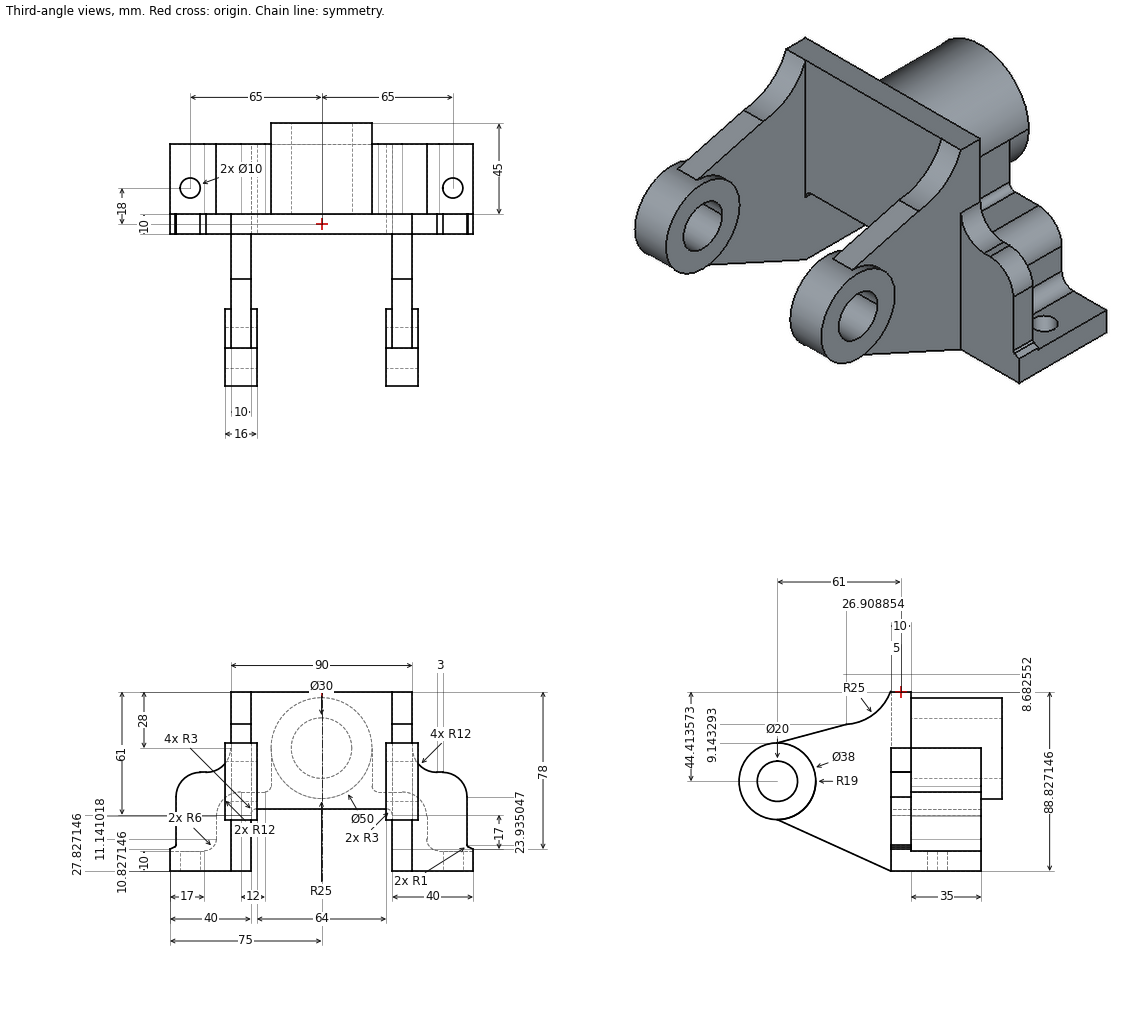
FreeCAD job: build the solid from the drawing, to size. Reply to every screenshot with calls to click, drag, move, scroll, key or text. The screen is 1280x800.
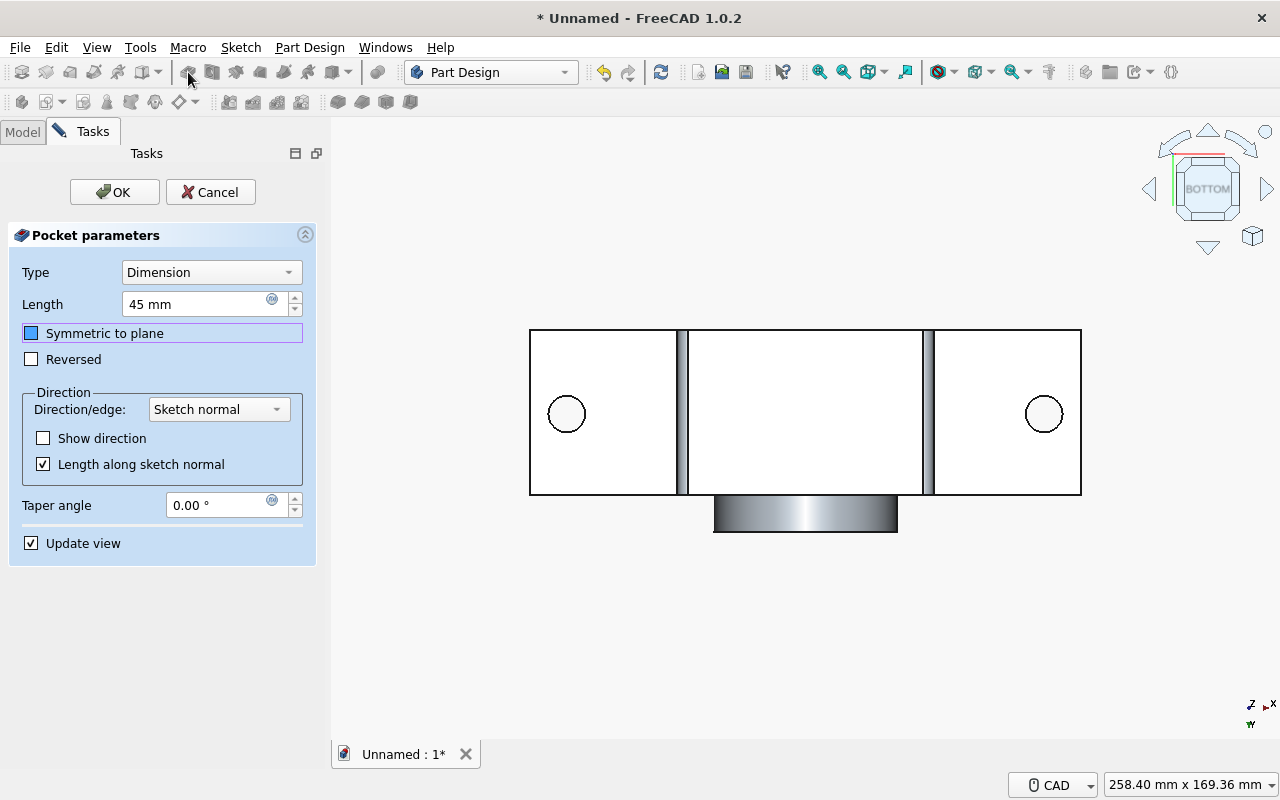
click(30, 333)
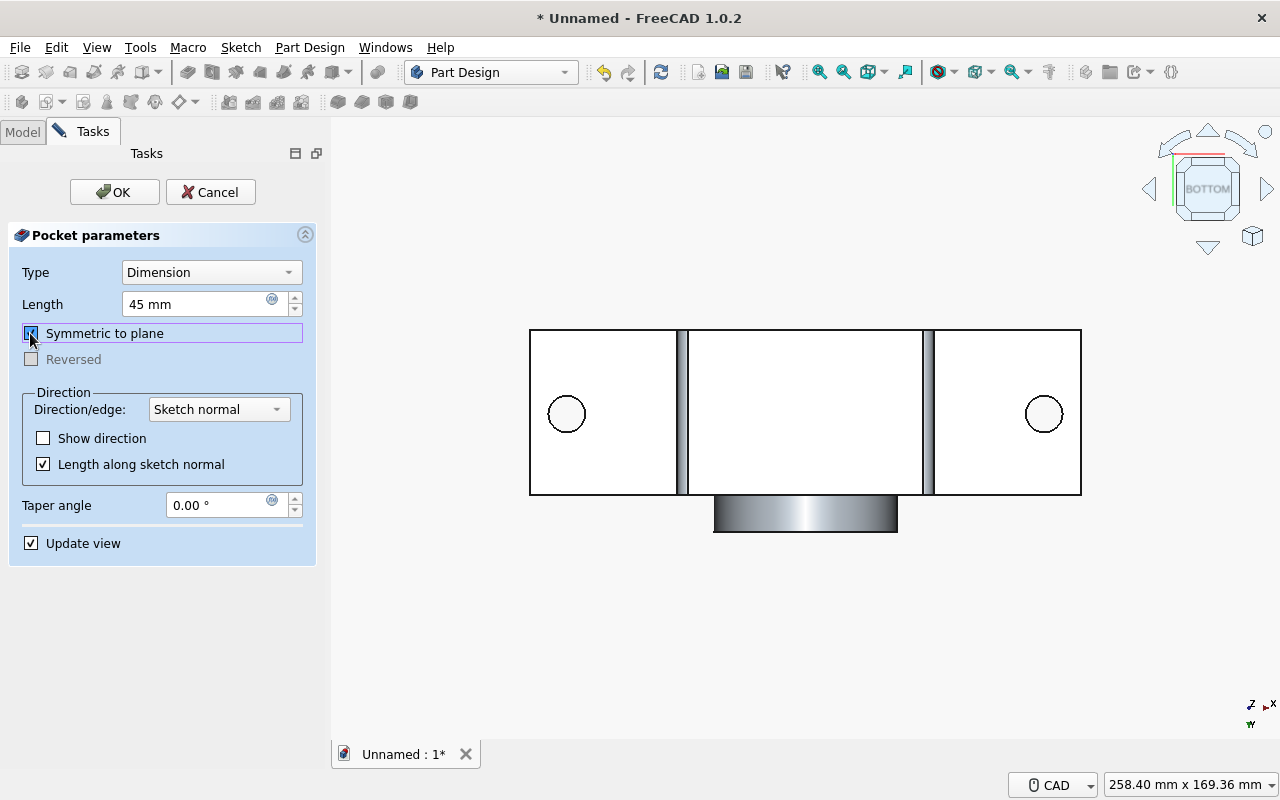
click(115, 192)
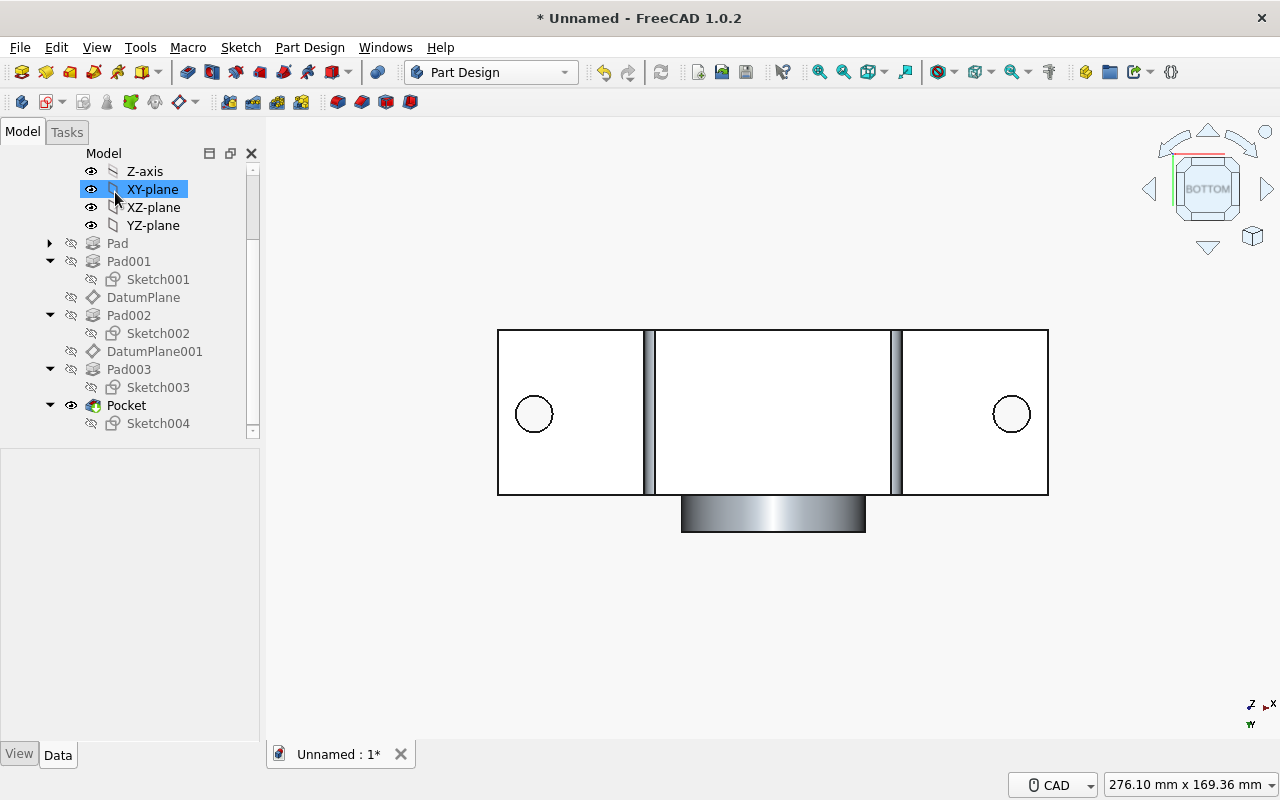
key(6)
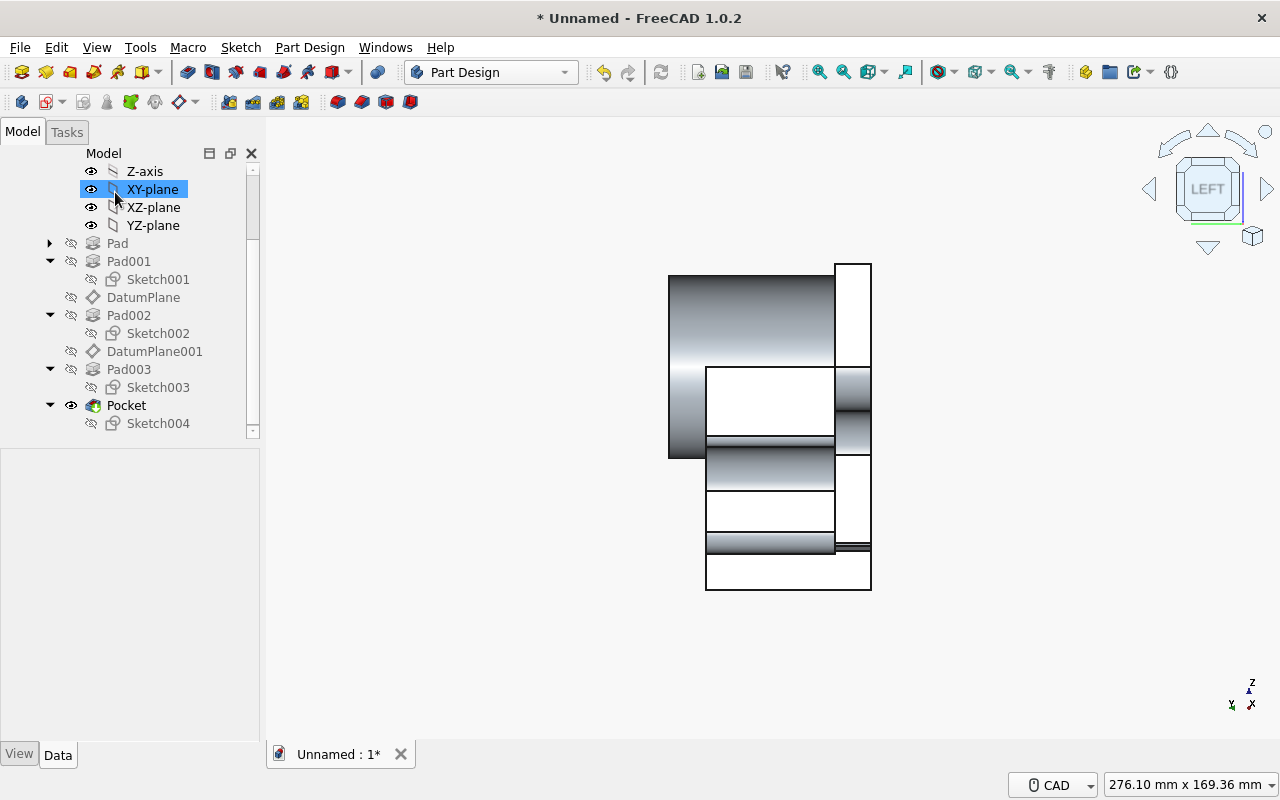
click(853, 285)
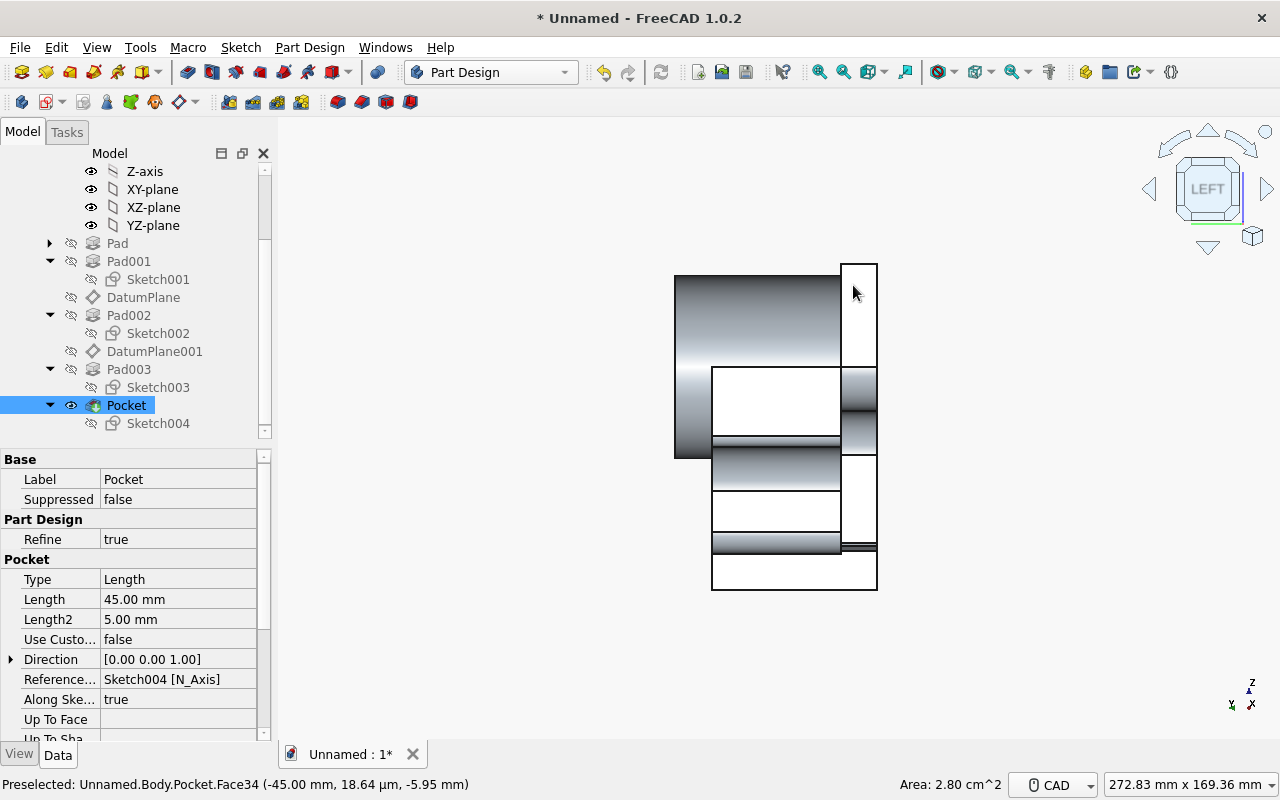
click(46, 102)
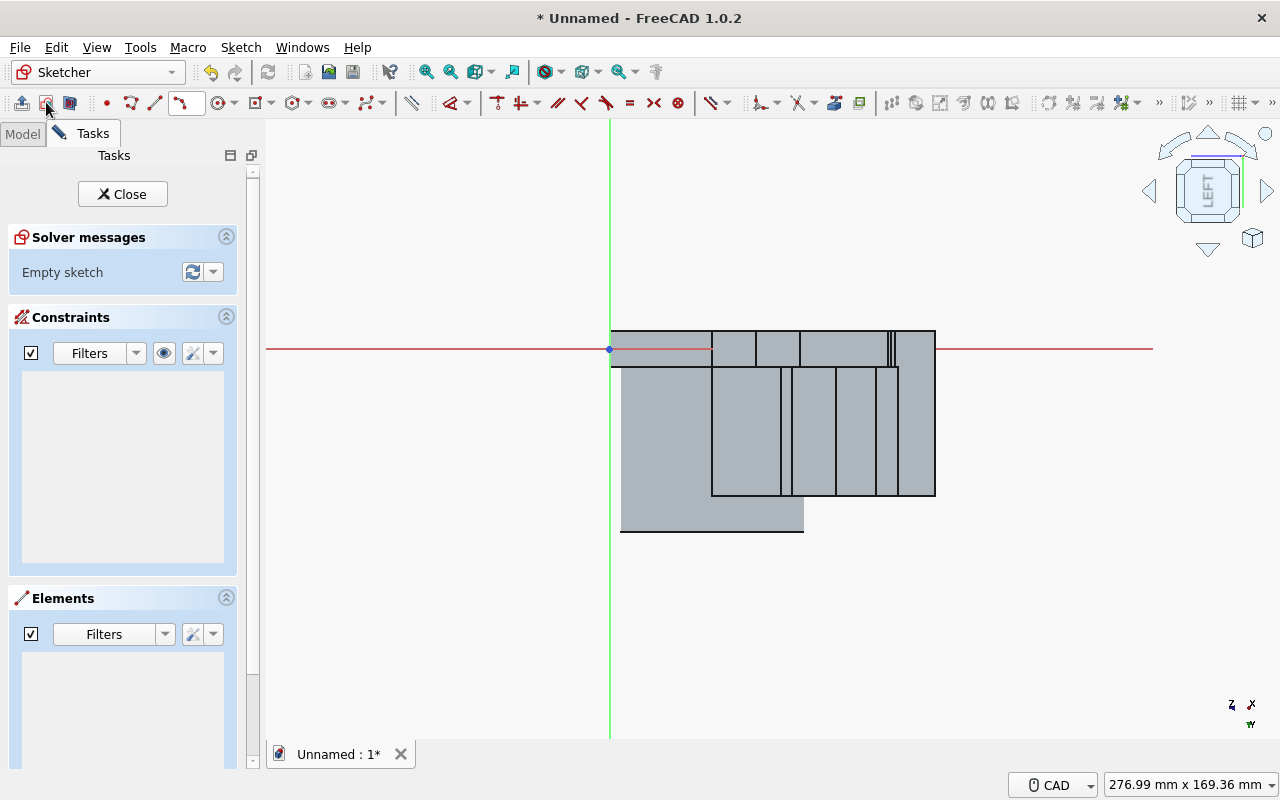
click(70, 104)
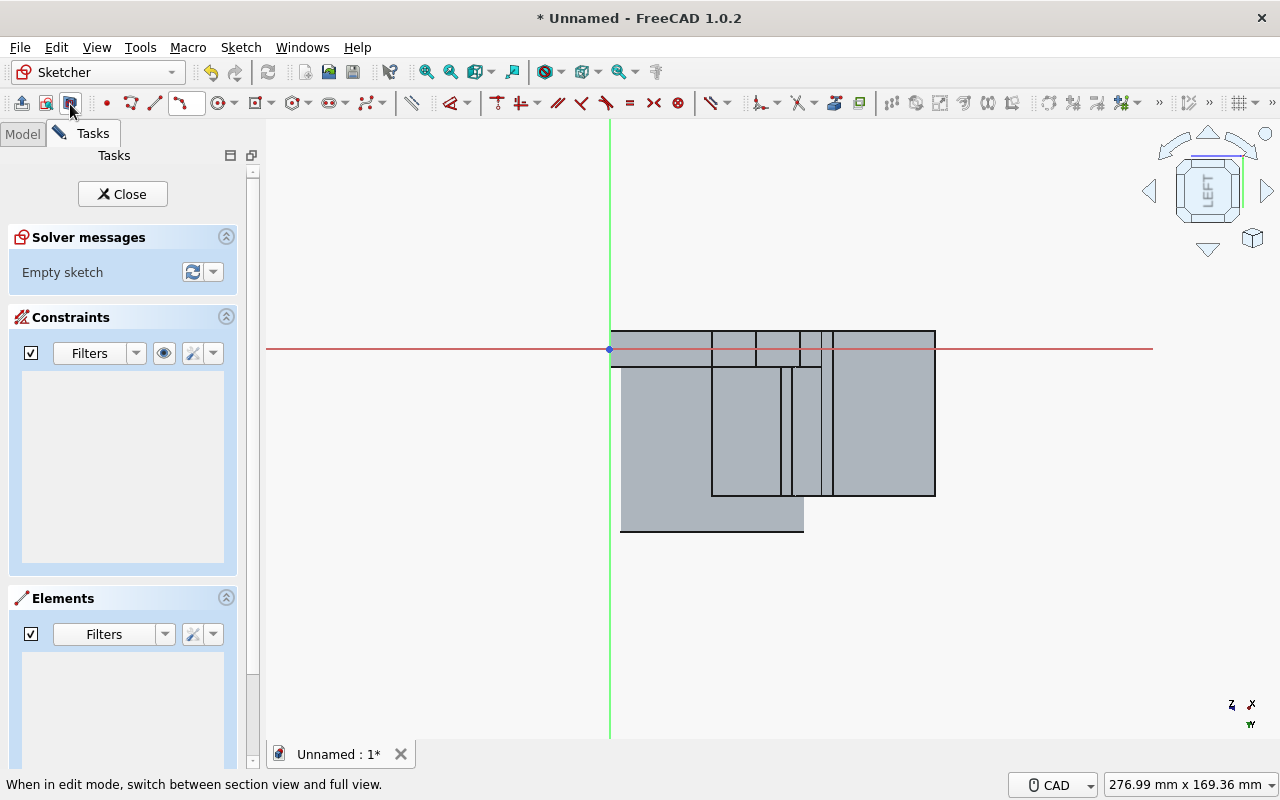
scroll(704, 429, down, 5)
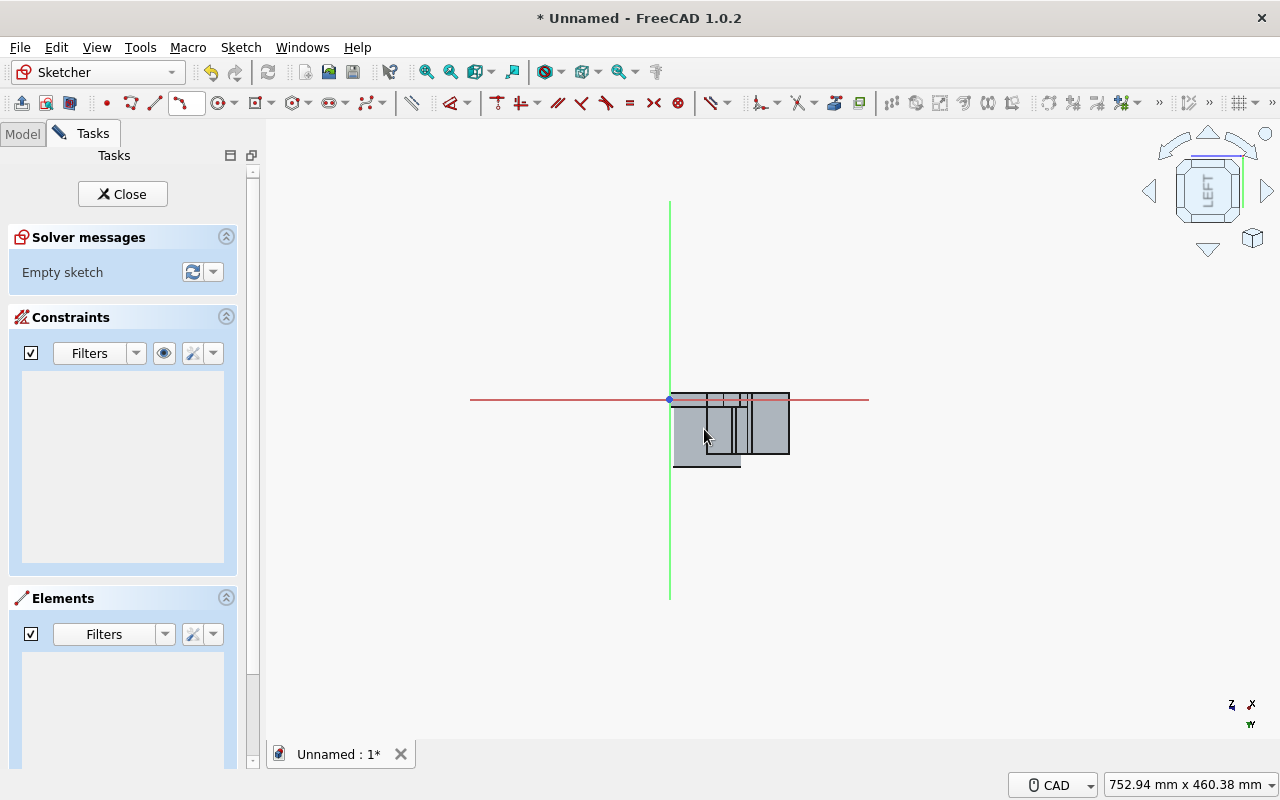
scroll(736, 341, up, 8)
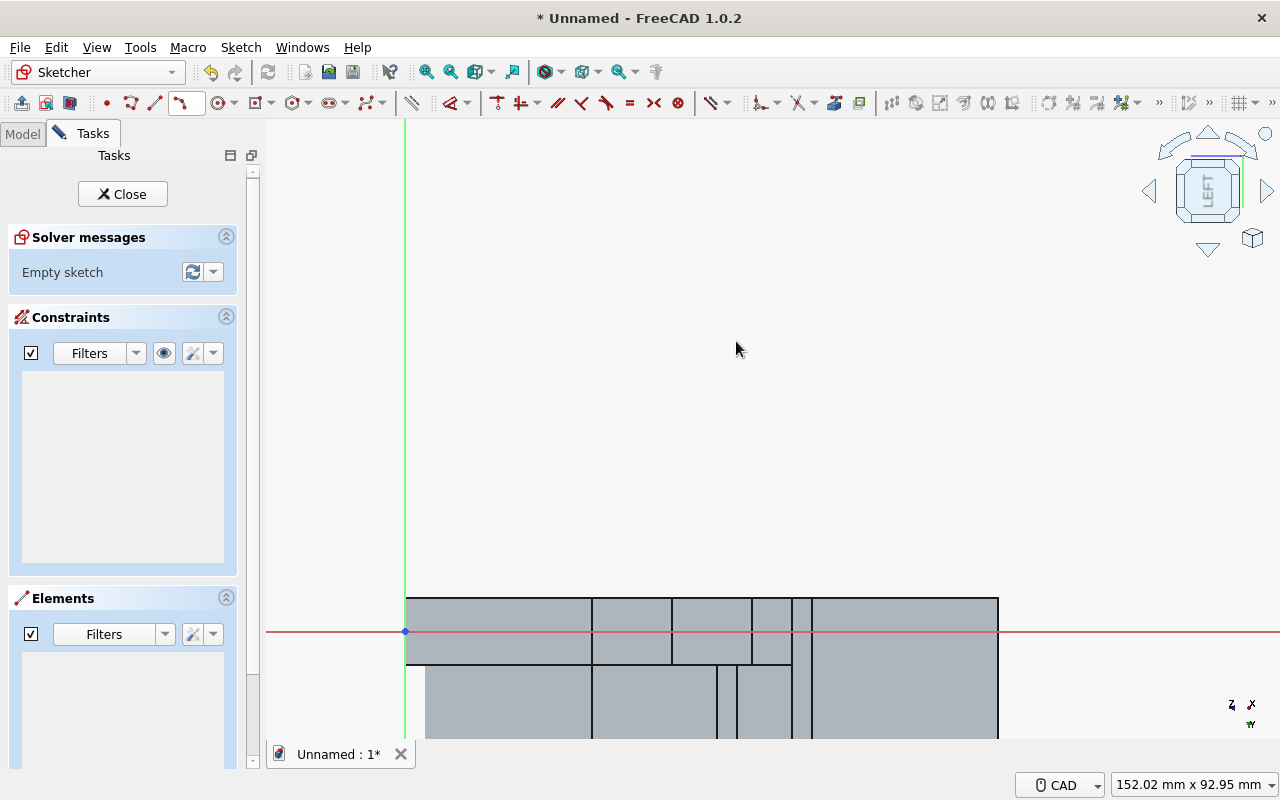
click(156, 104)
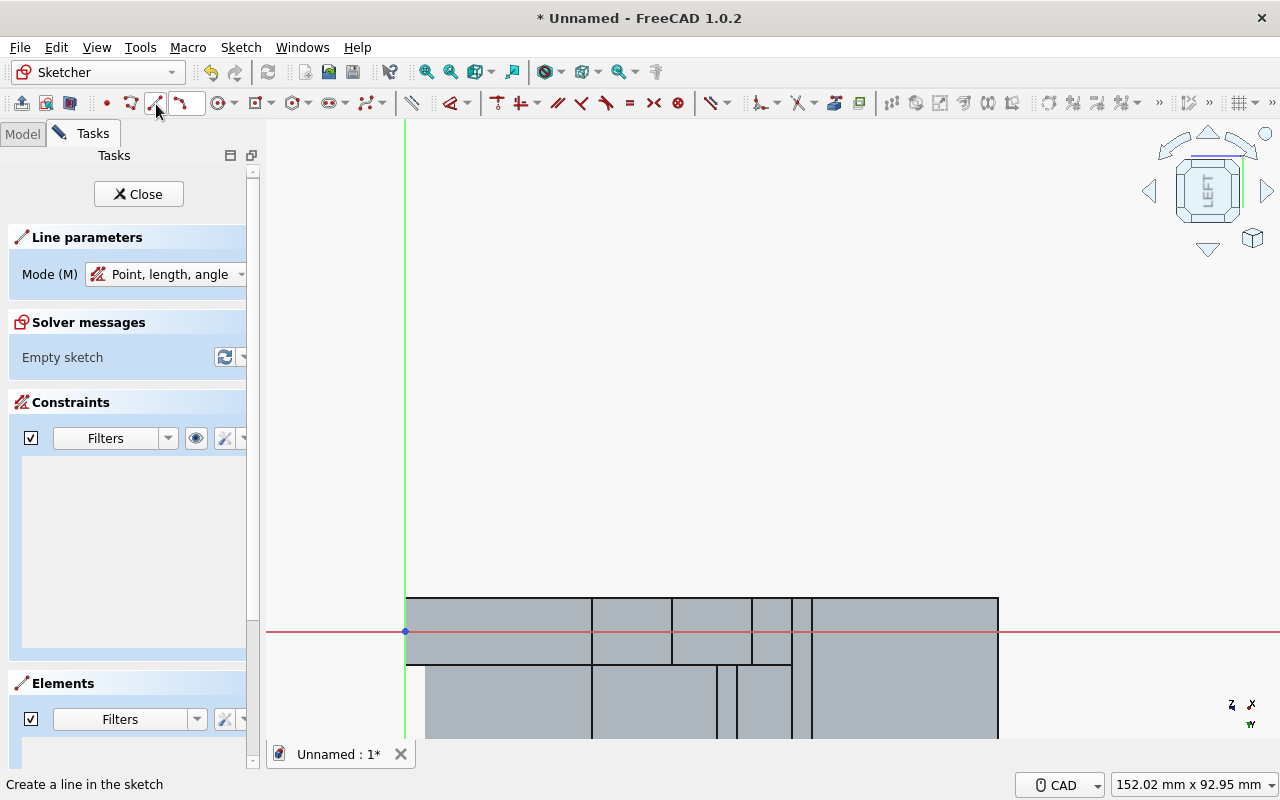
click(575, 225)
click(514, 452)